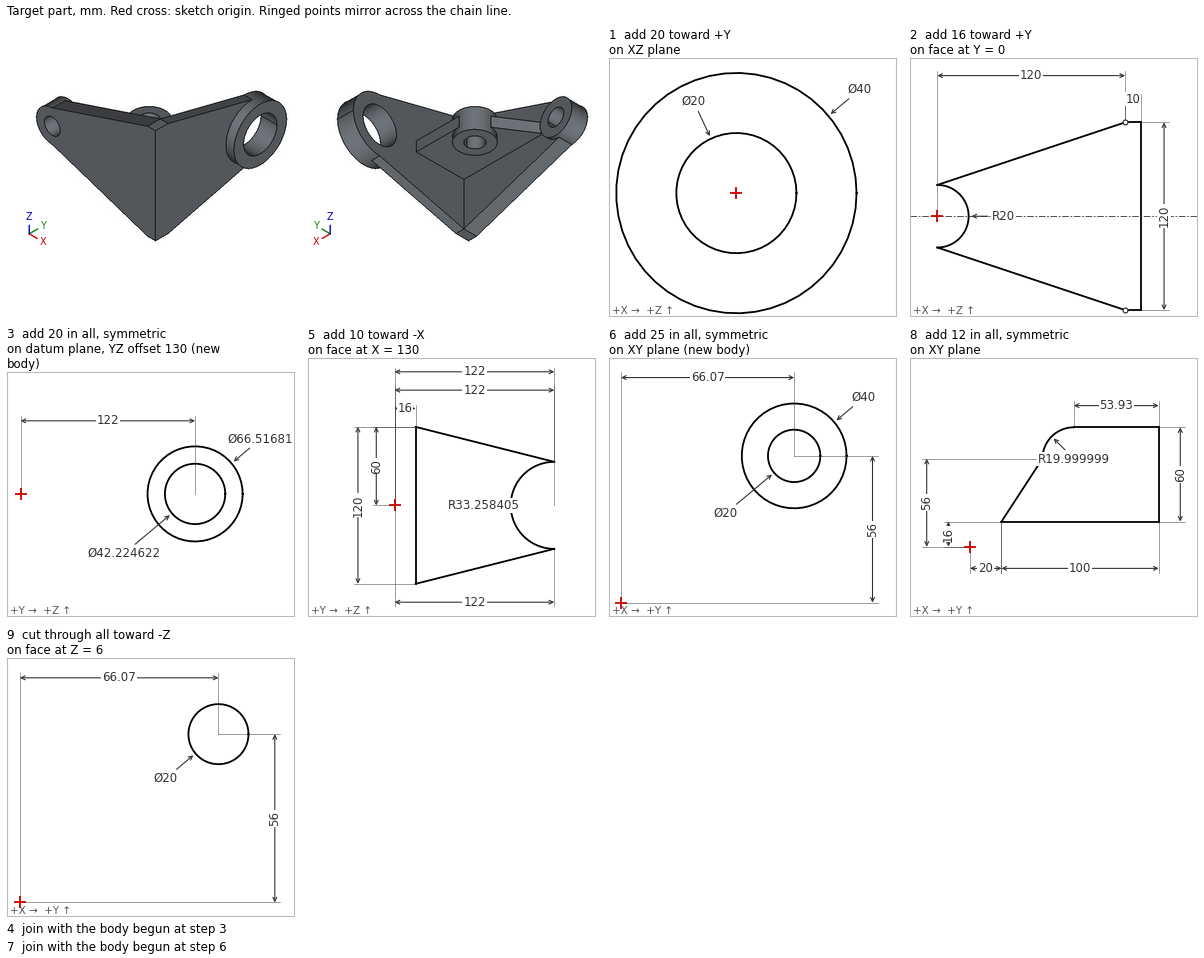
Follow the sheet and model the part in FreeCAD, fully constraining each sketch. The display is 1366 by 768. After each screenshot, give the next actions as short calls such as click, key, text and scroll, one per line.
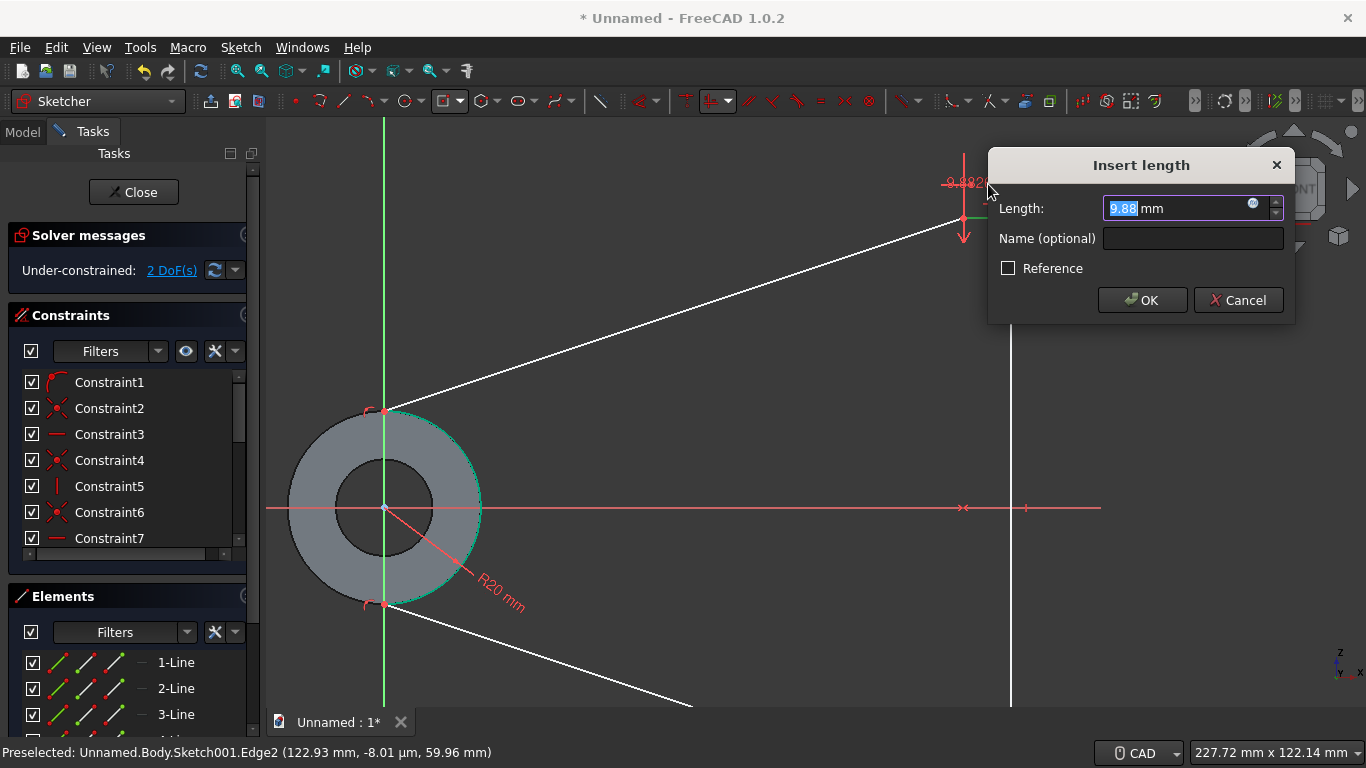
text(10)
key(Return)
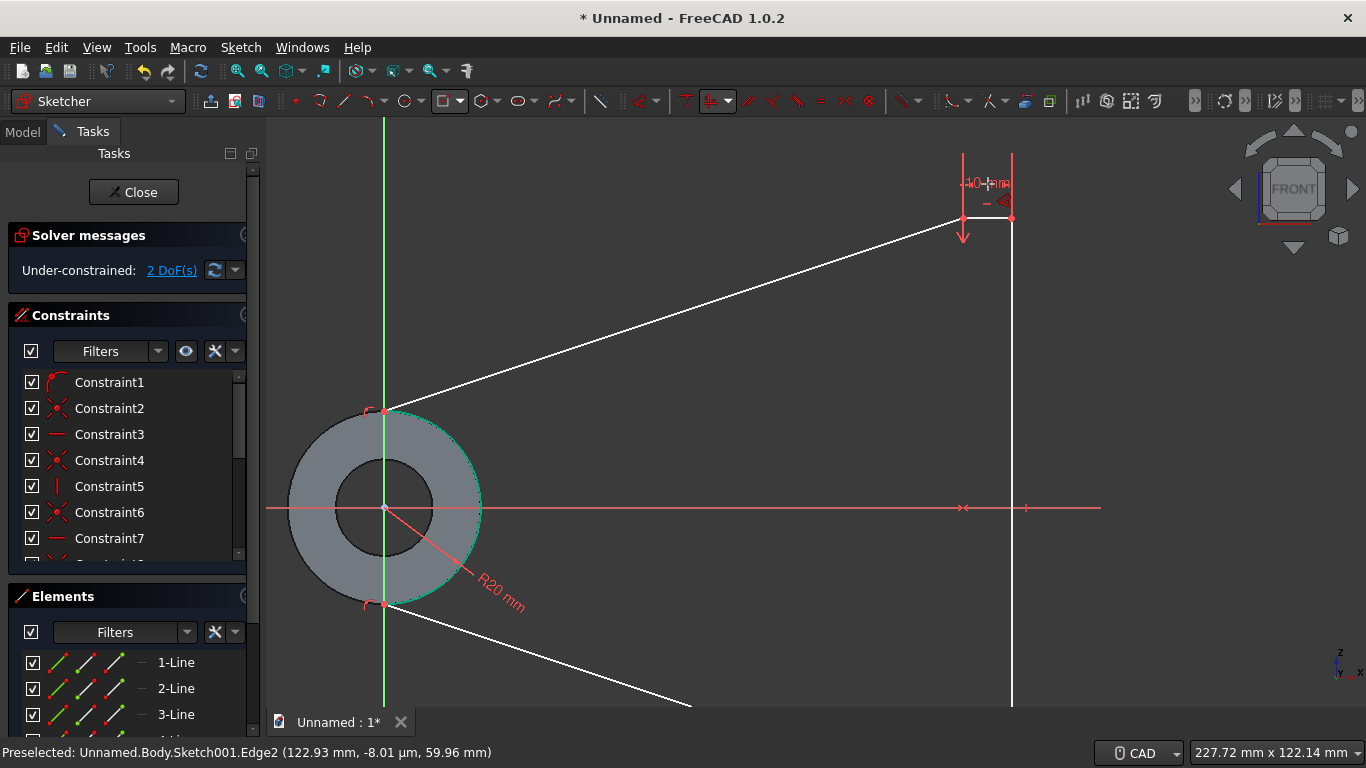
click(1012, 392)
click(1046, 449)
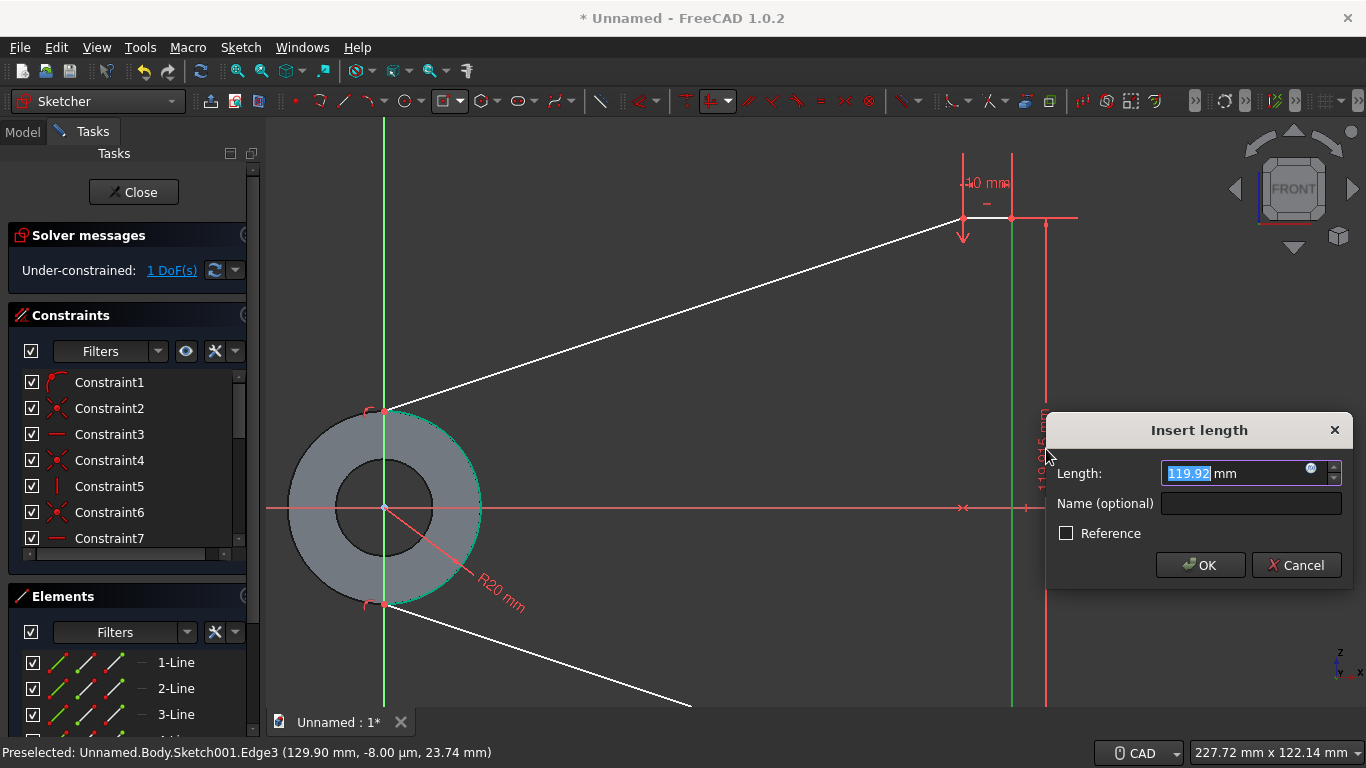
text(120)
key(Return)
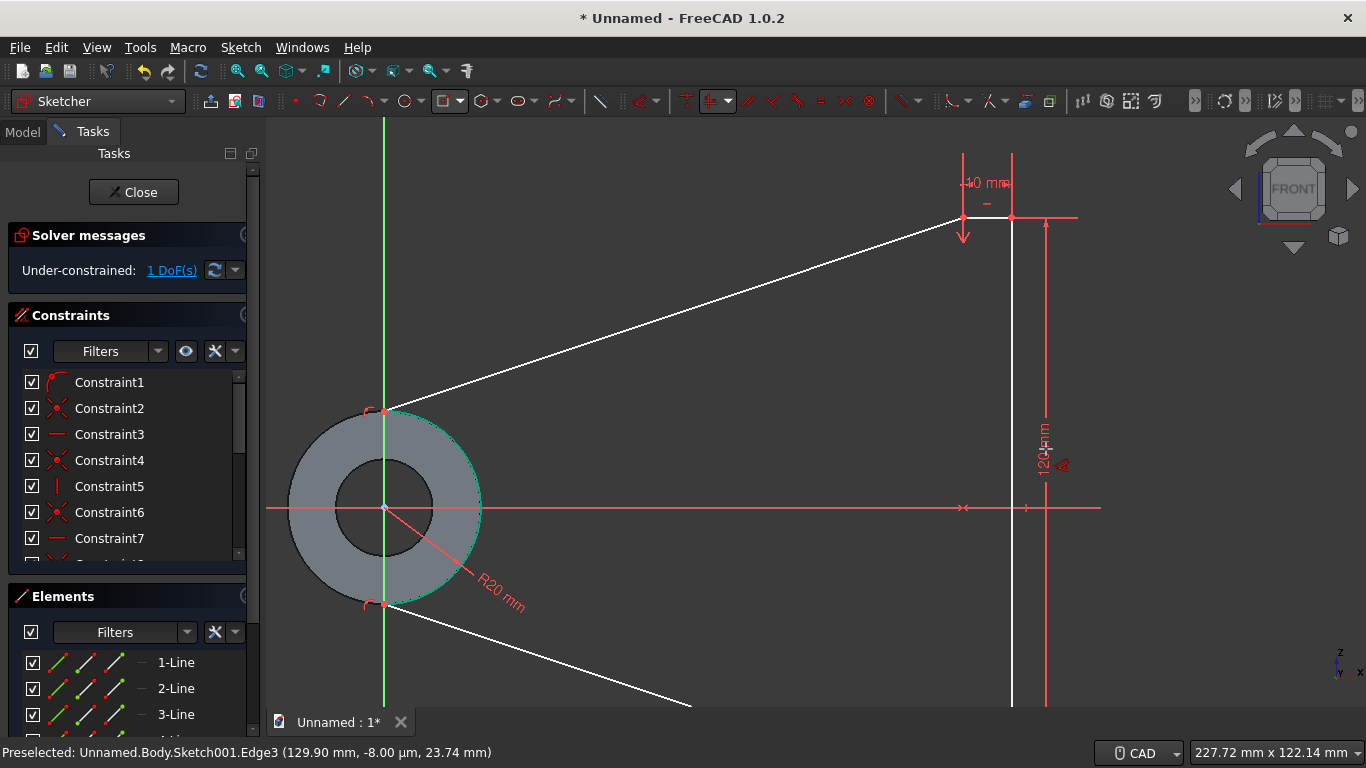
click(963, 218)
click(674, 184)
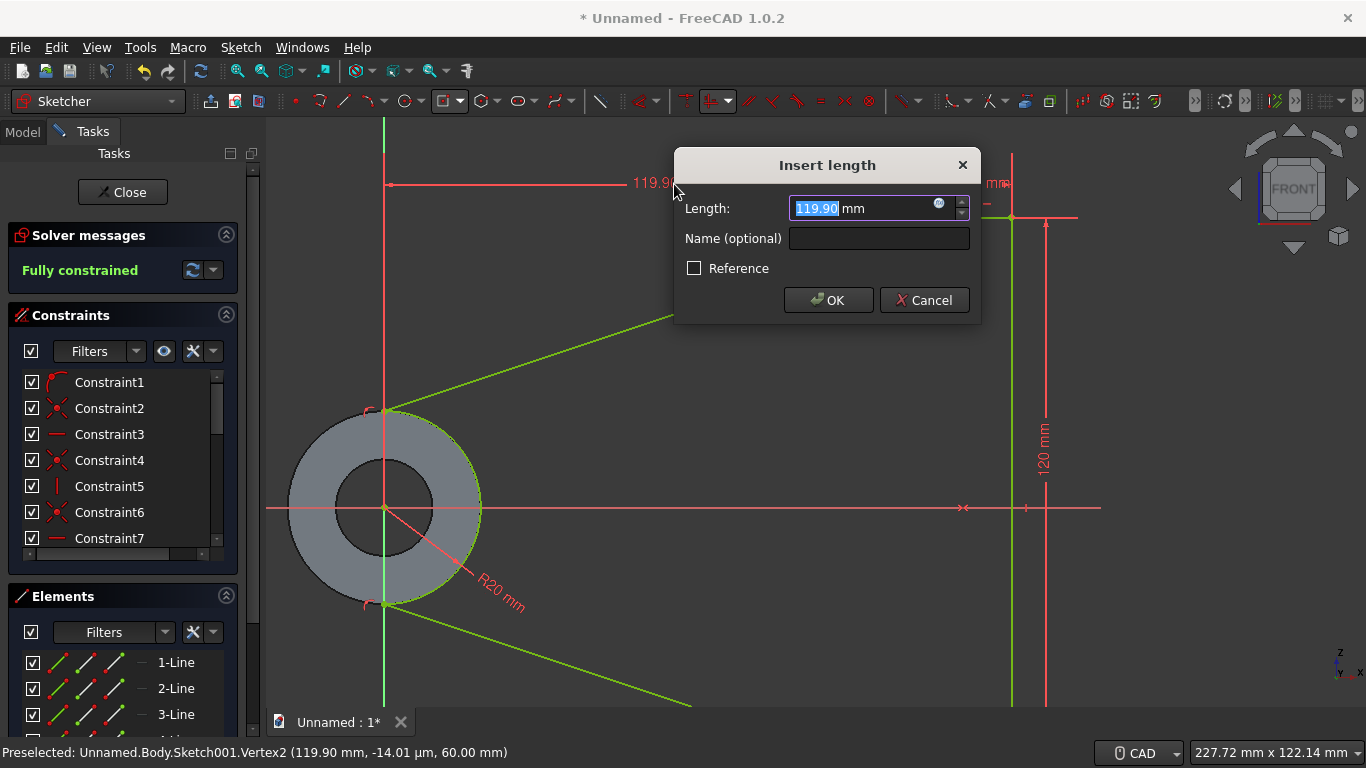
text(120)
key(Return)
key(Escape)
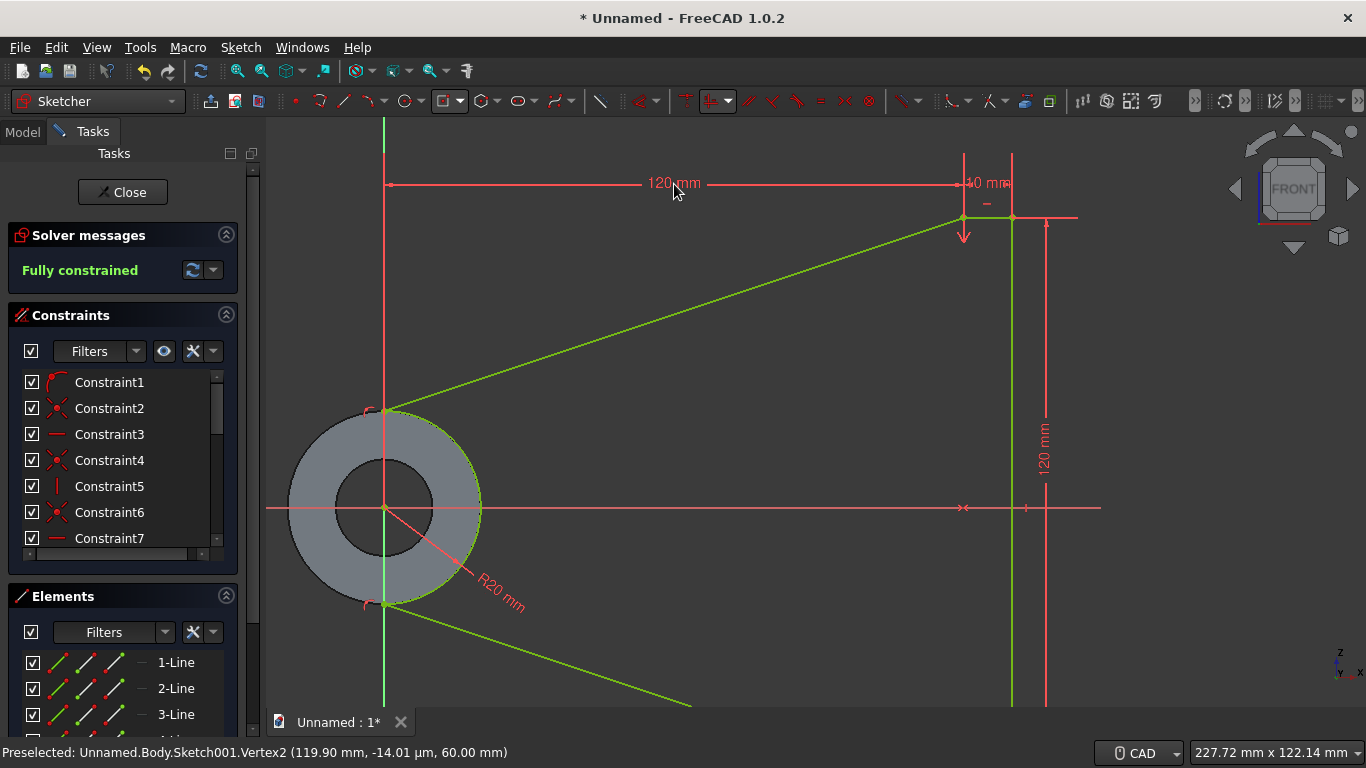
click(123, 192)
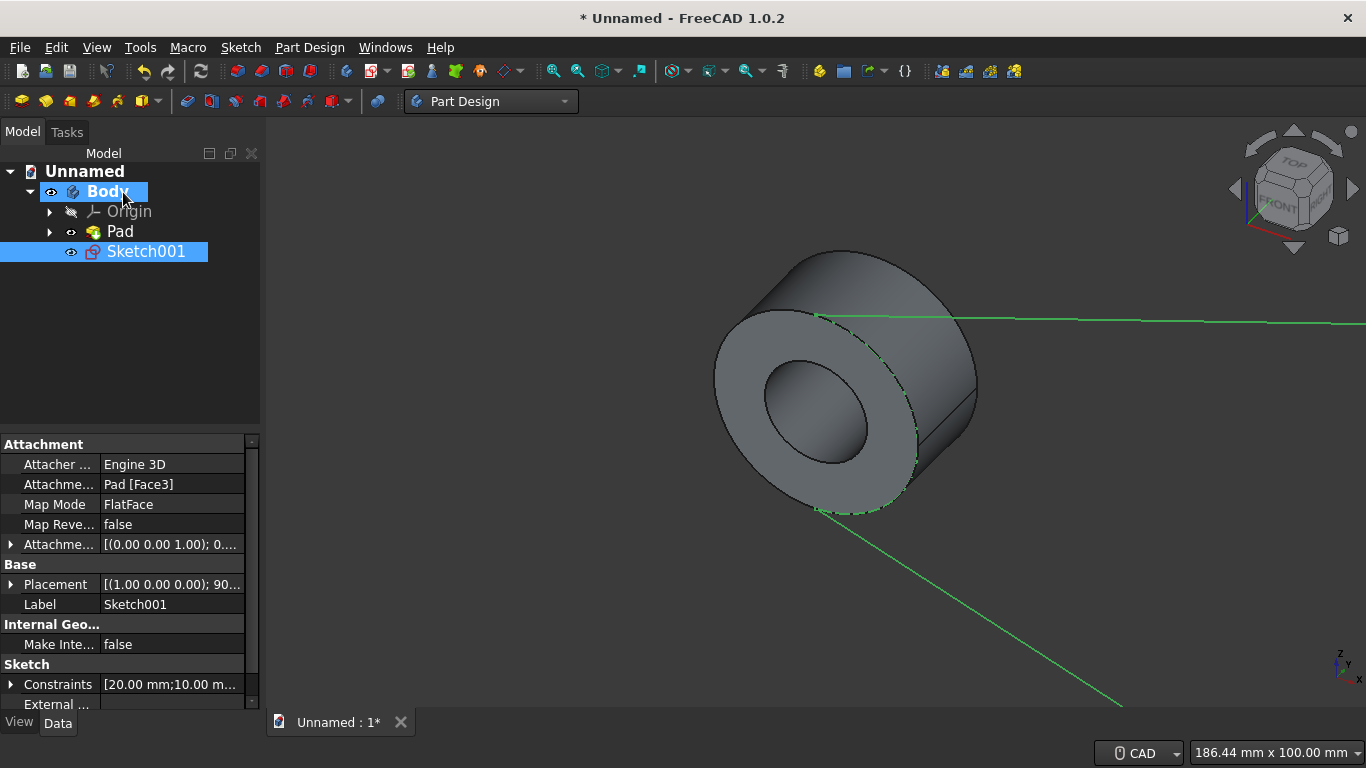
click(22, 102)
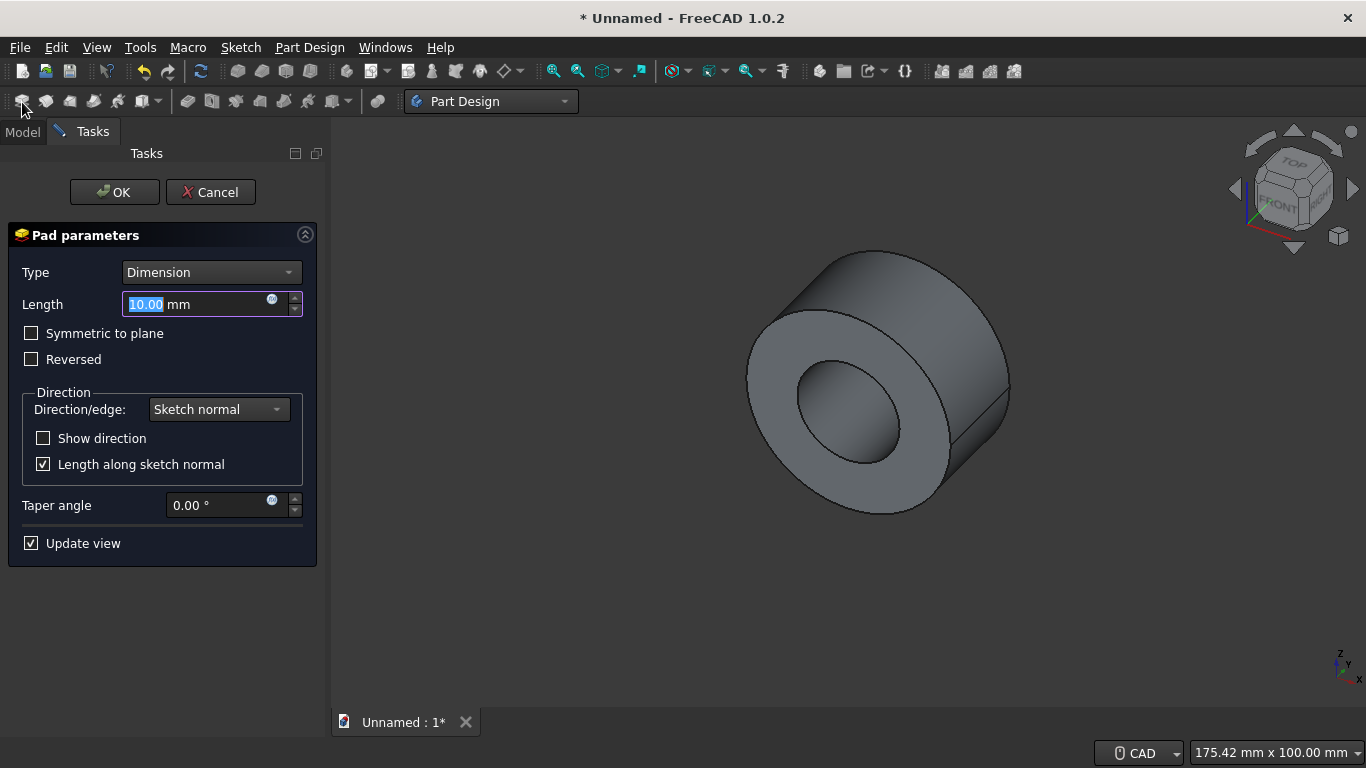
text(16)
key(Tab)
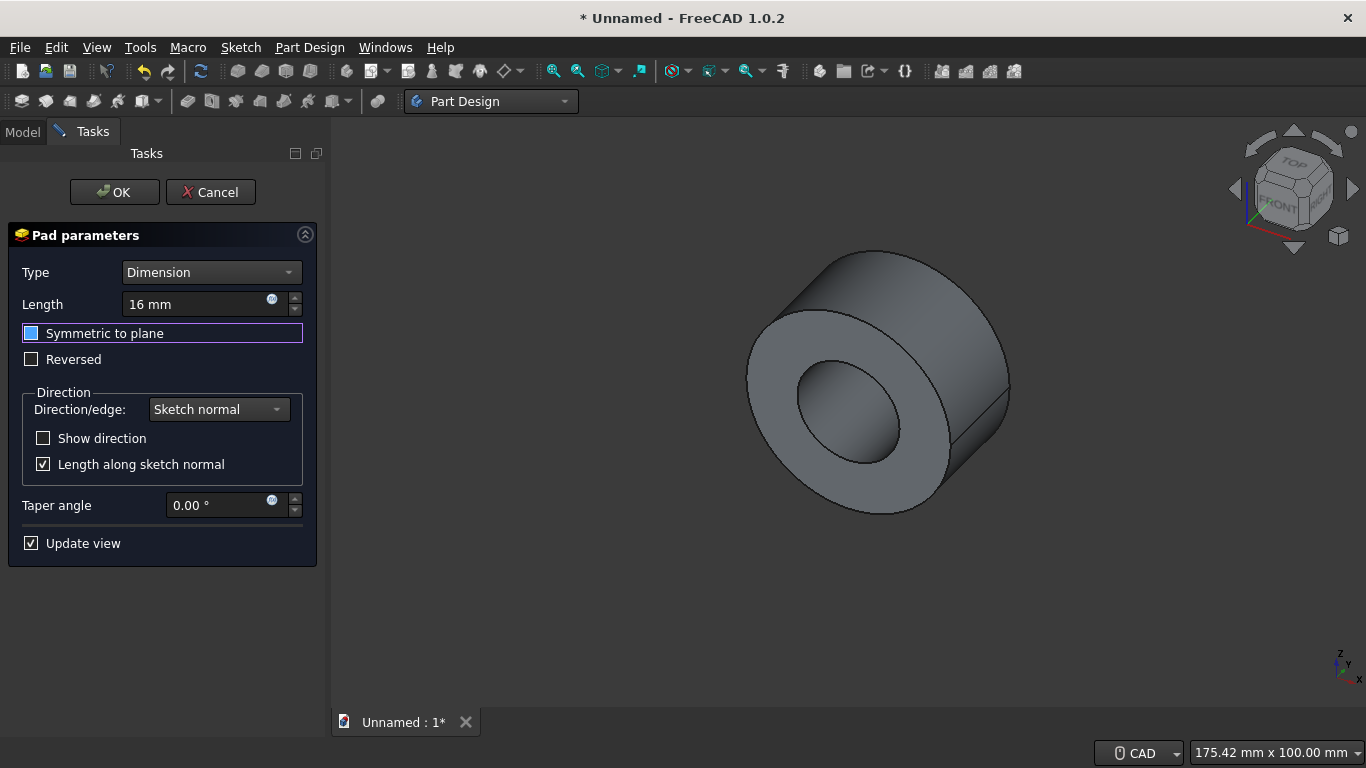
click(30, 359)